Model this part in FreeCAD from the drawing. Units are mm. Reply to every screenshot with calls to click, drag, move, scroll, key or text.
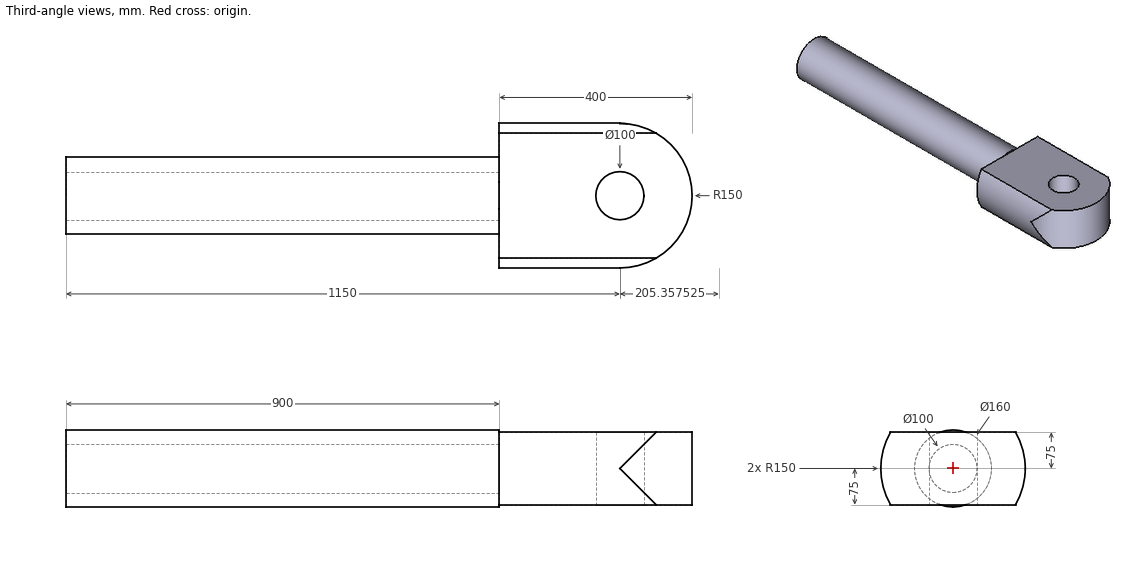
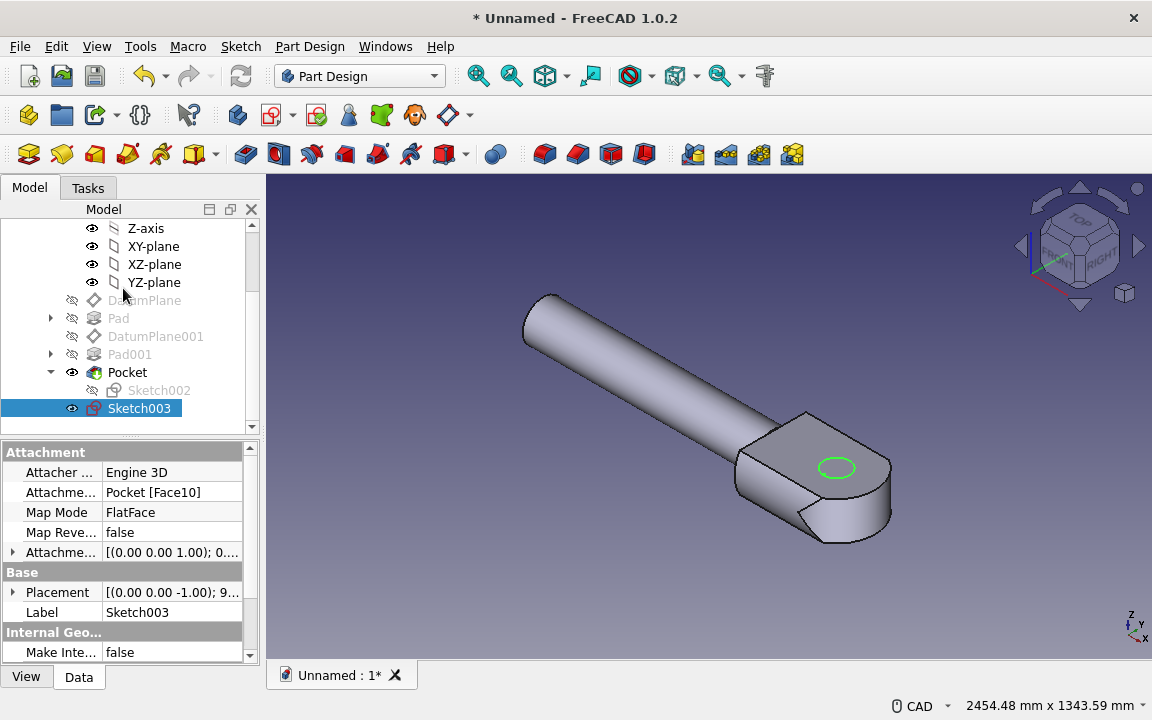
click(246, 154)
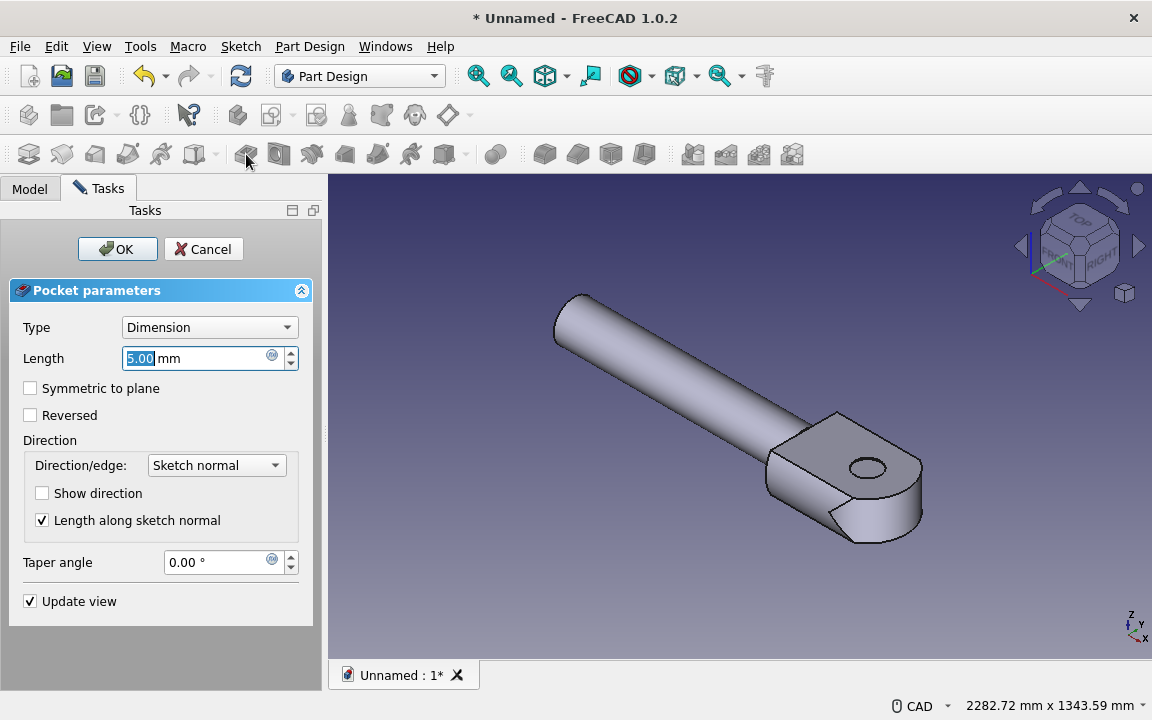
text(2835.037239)
key(Tab)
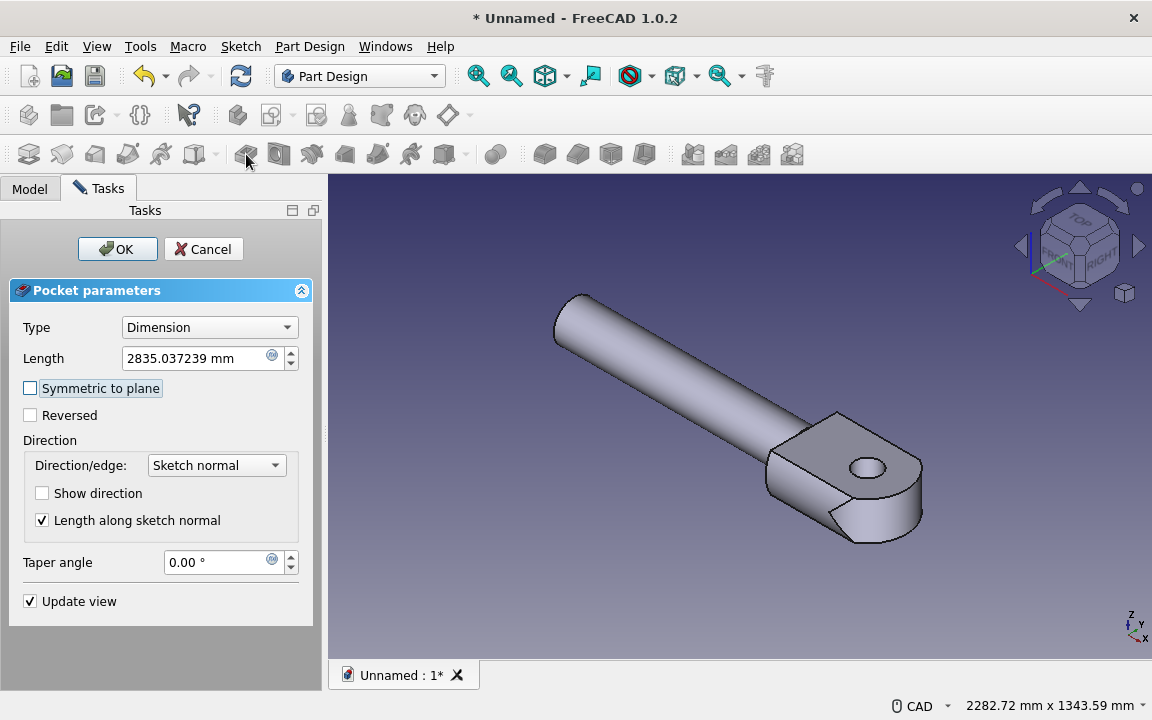
click(31, 388)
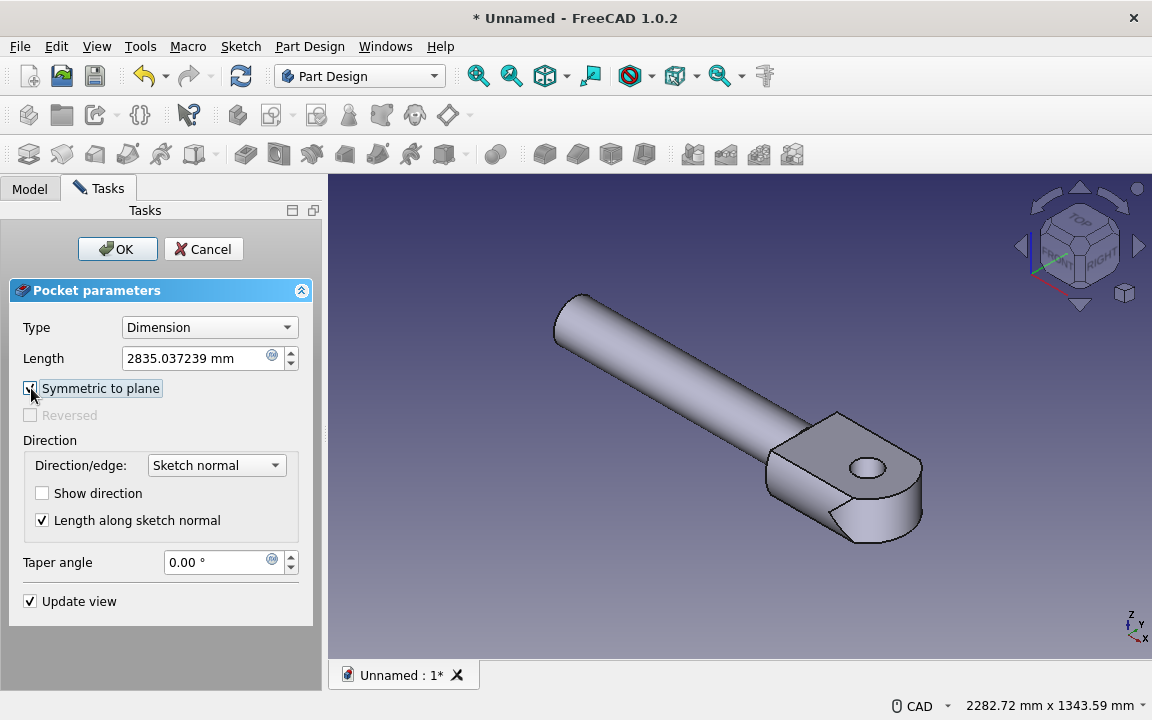
click(118, 249)